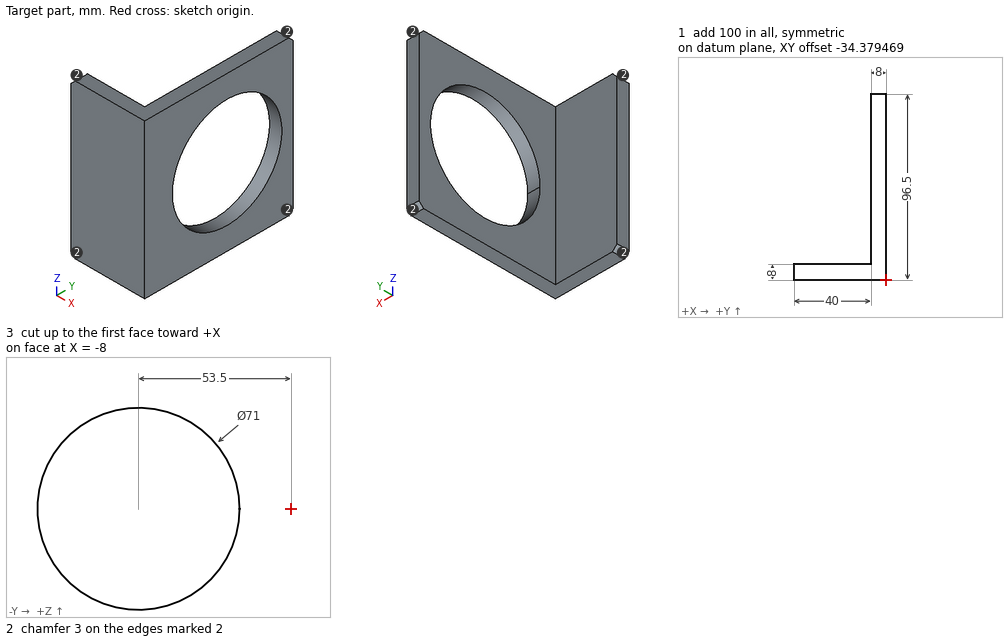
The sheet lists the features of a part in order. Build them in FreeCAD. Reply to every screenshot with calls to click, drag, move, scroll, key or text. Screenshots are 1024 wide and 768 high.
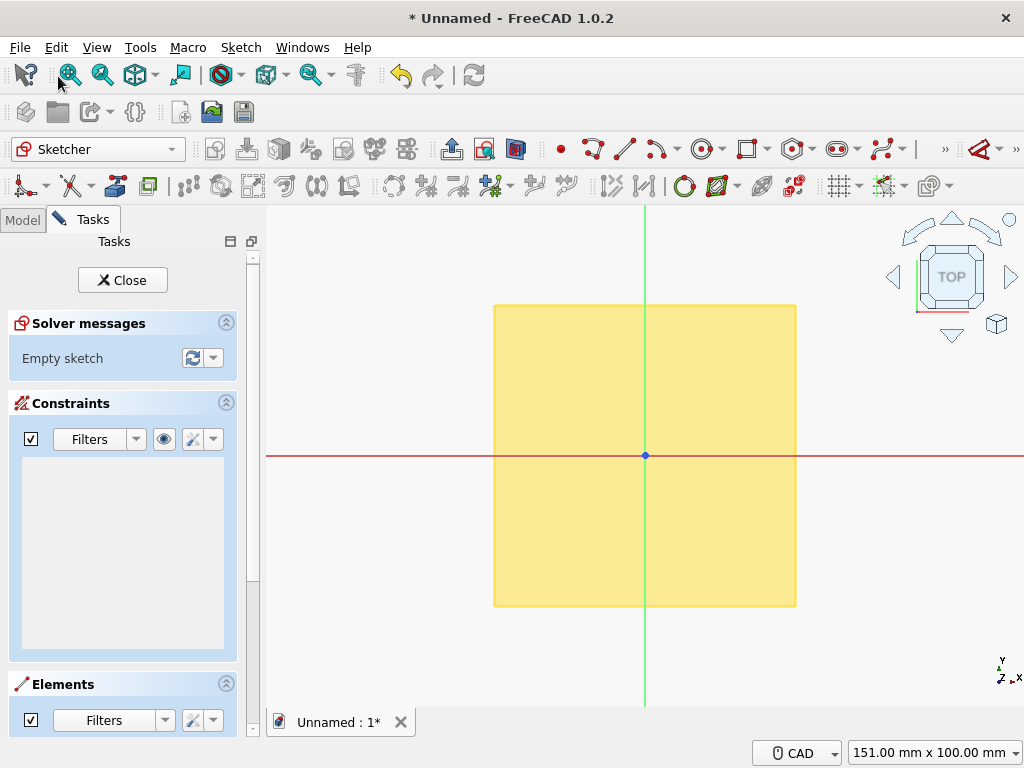
scroll(640, 679, down, 3)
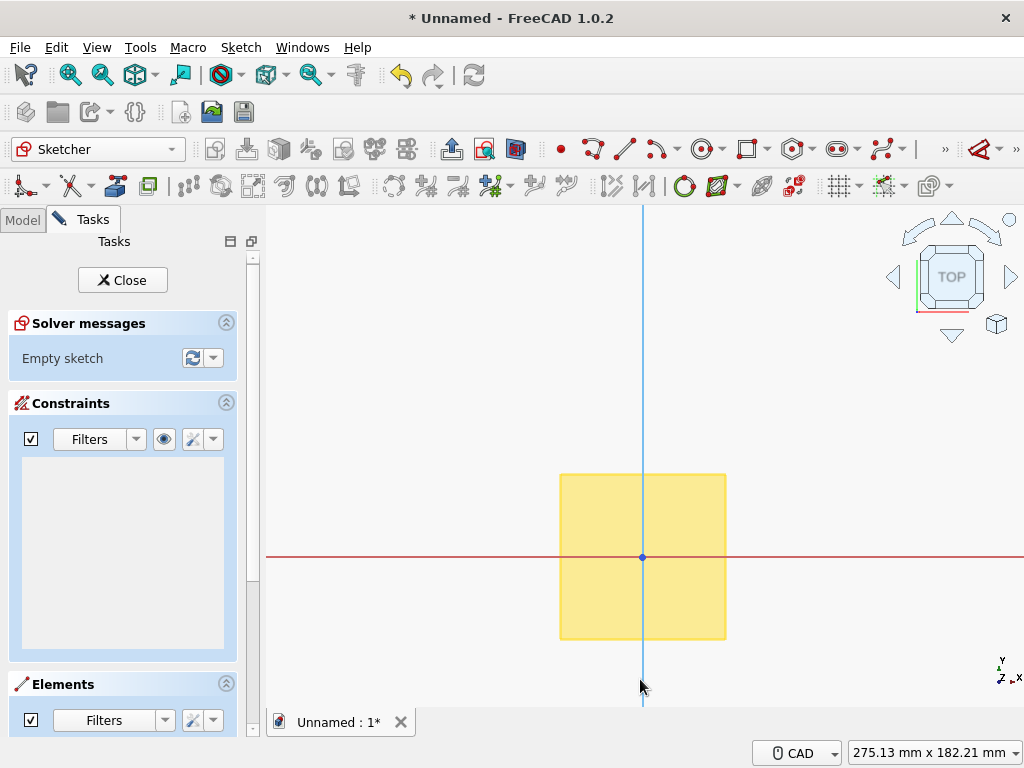
key(g)
key(m)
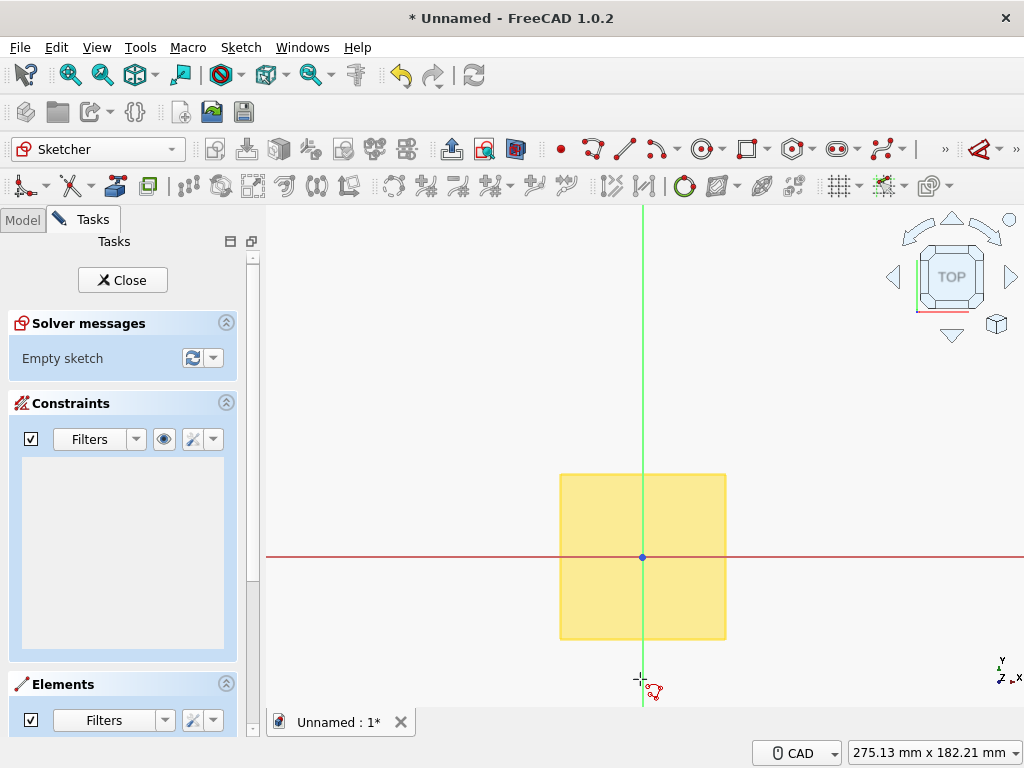
click(643, 557)
click(634, 291)
click(621, 291)
click(621, 535)
click(511, 535)
click(511, 548)
click(643, 557)
key(Escape)
key(Escape)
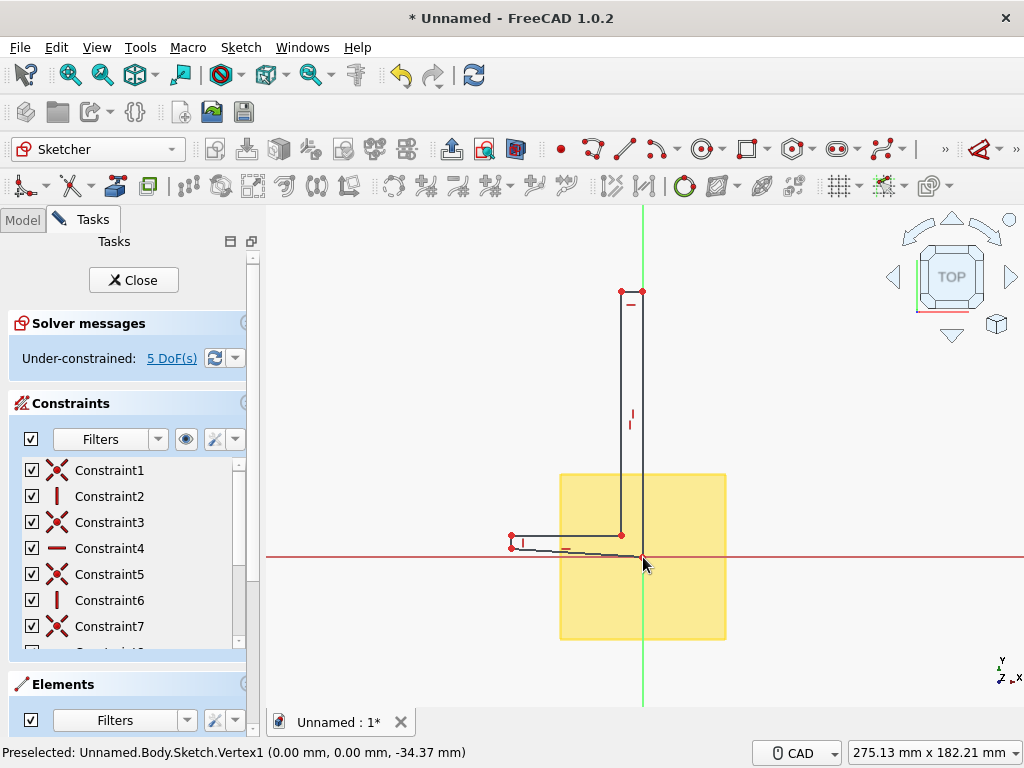
click(603, 555)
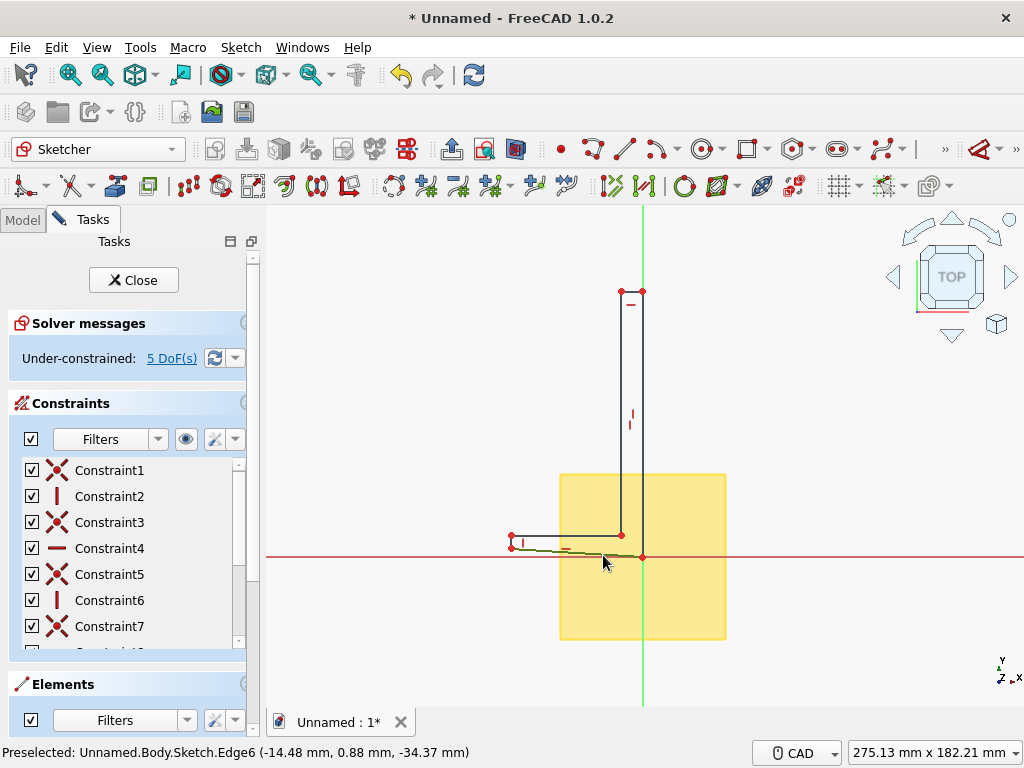
key(h)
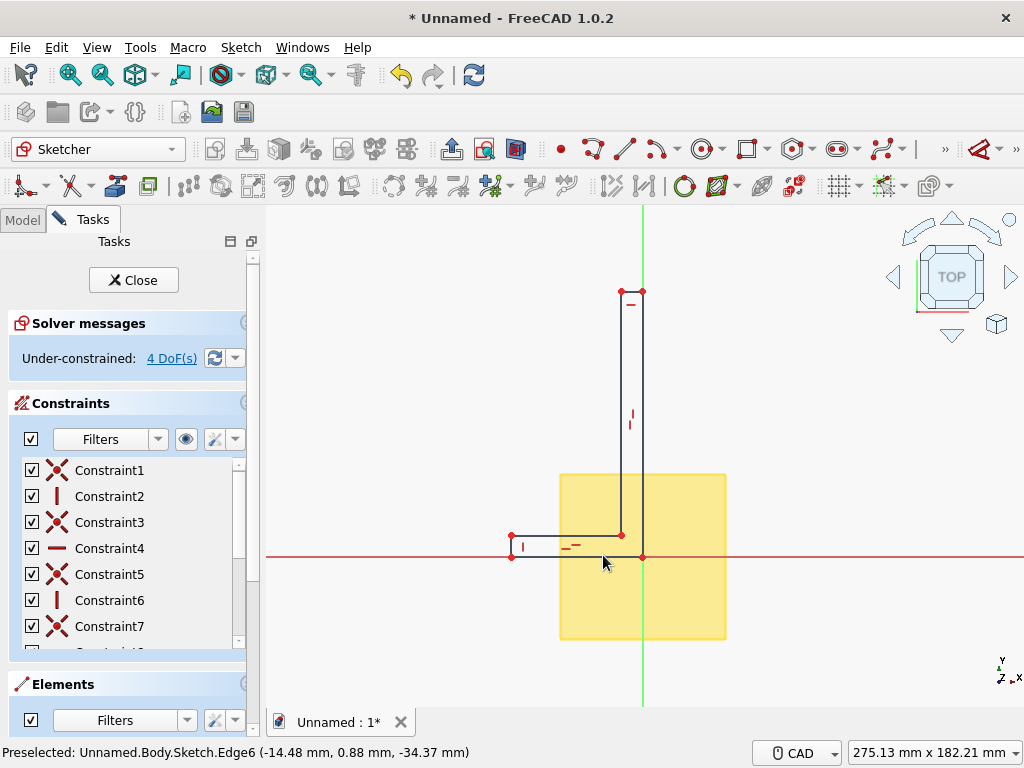
click(980, 150)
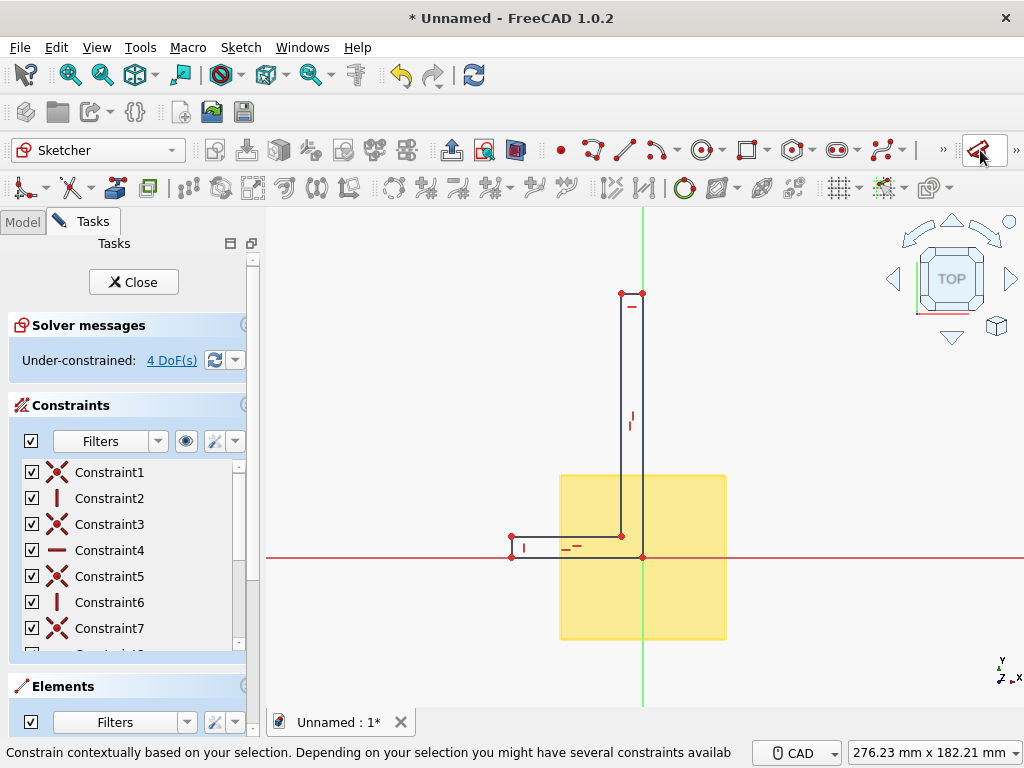
scroll(632, 294, up, 3)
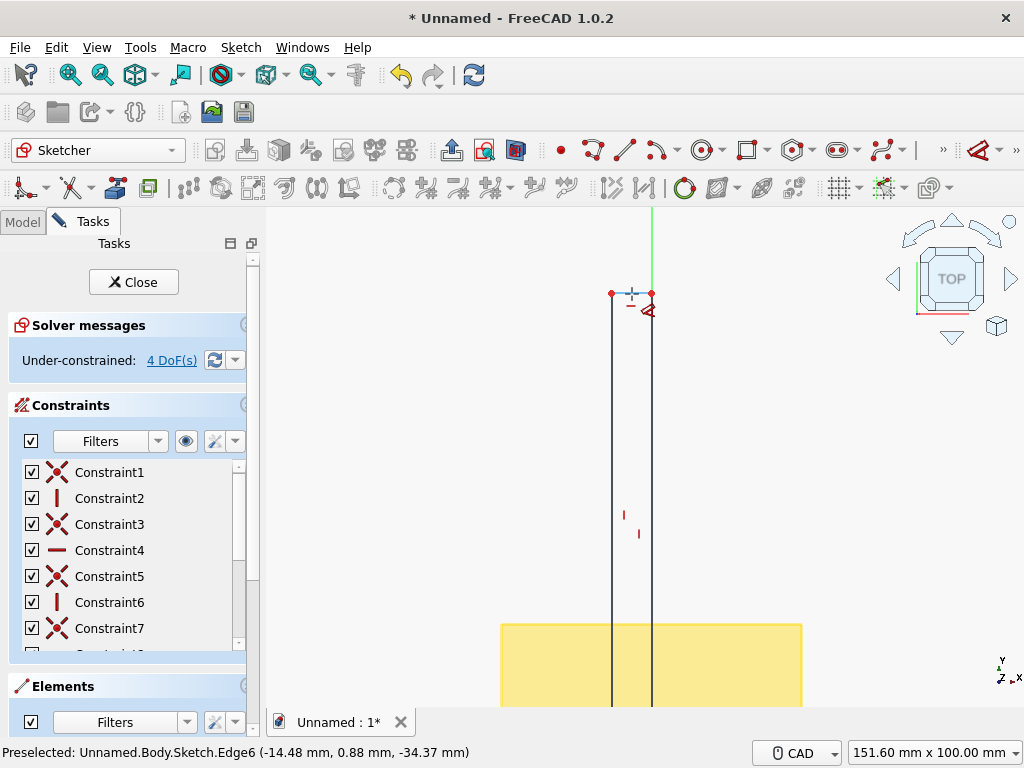
click(632, 293)
click(632, 259)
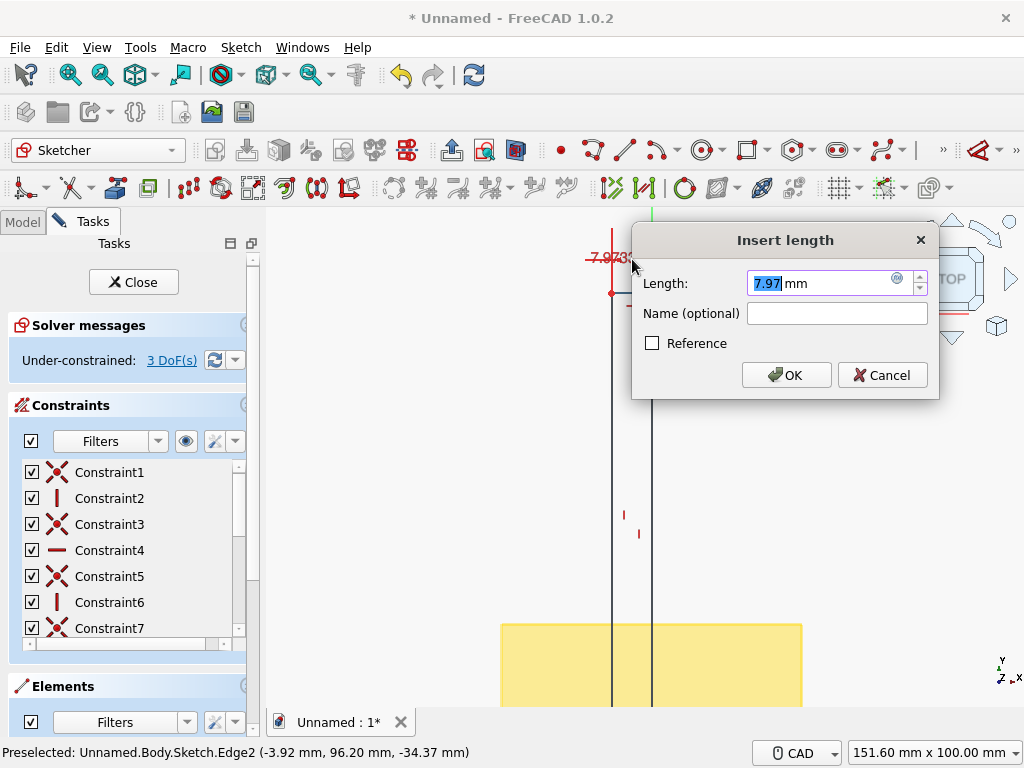
text(8)
key(Return)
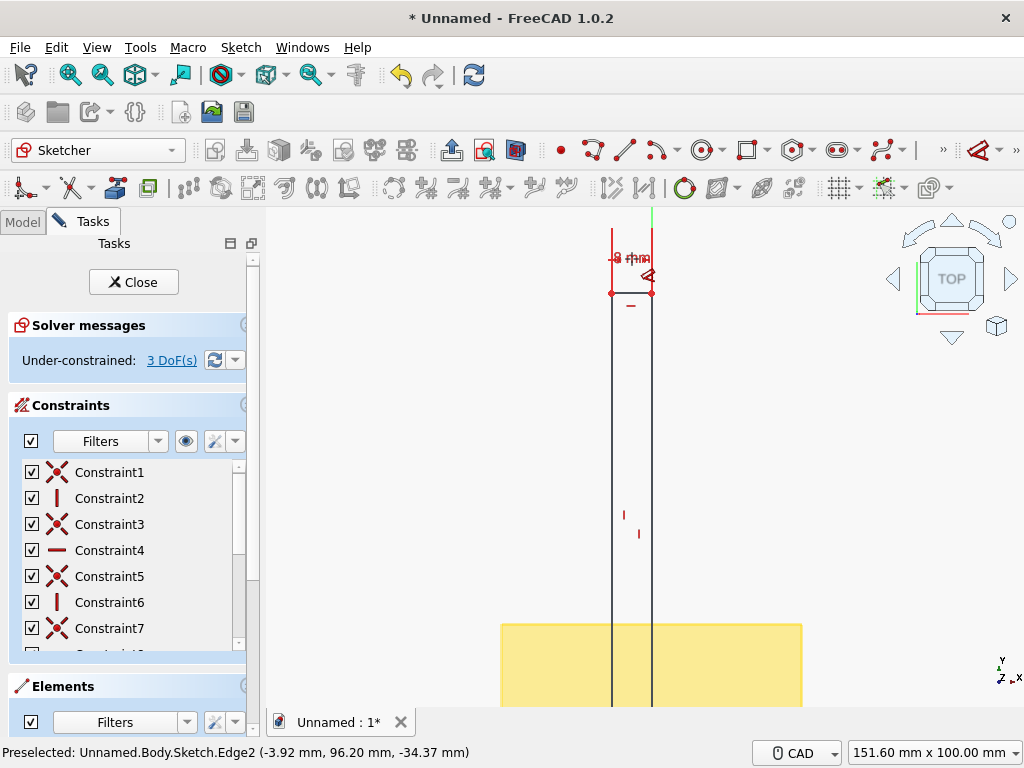
scroll(668, 302, down, 2)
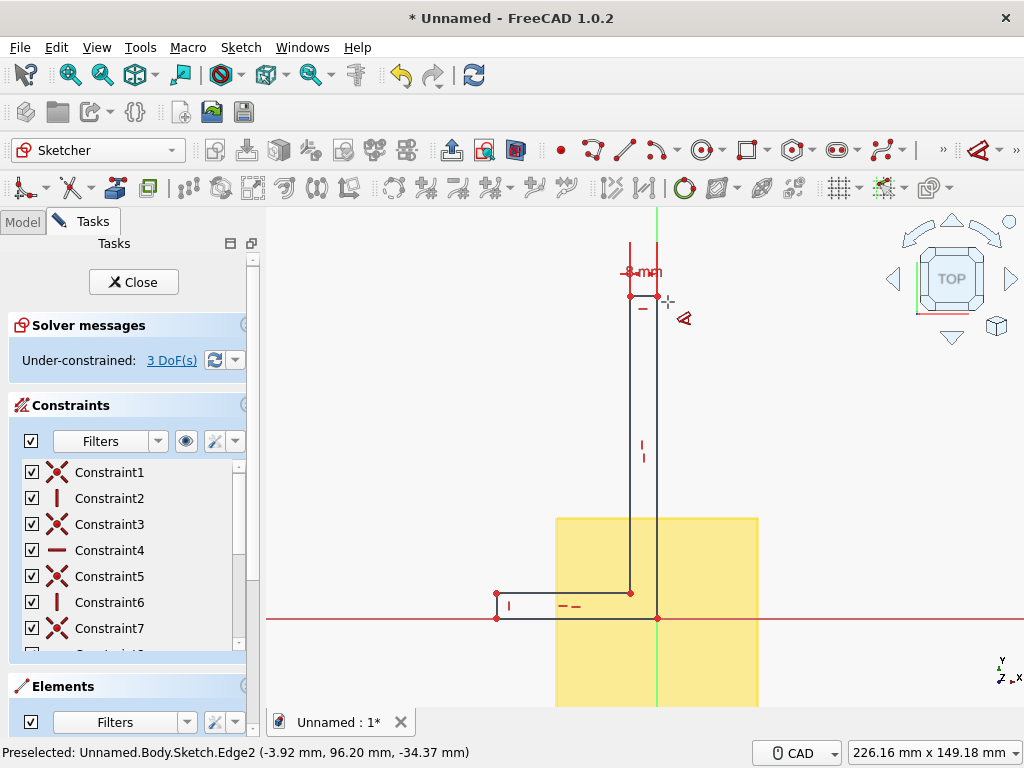
scroll(497, 601, up, 3)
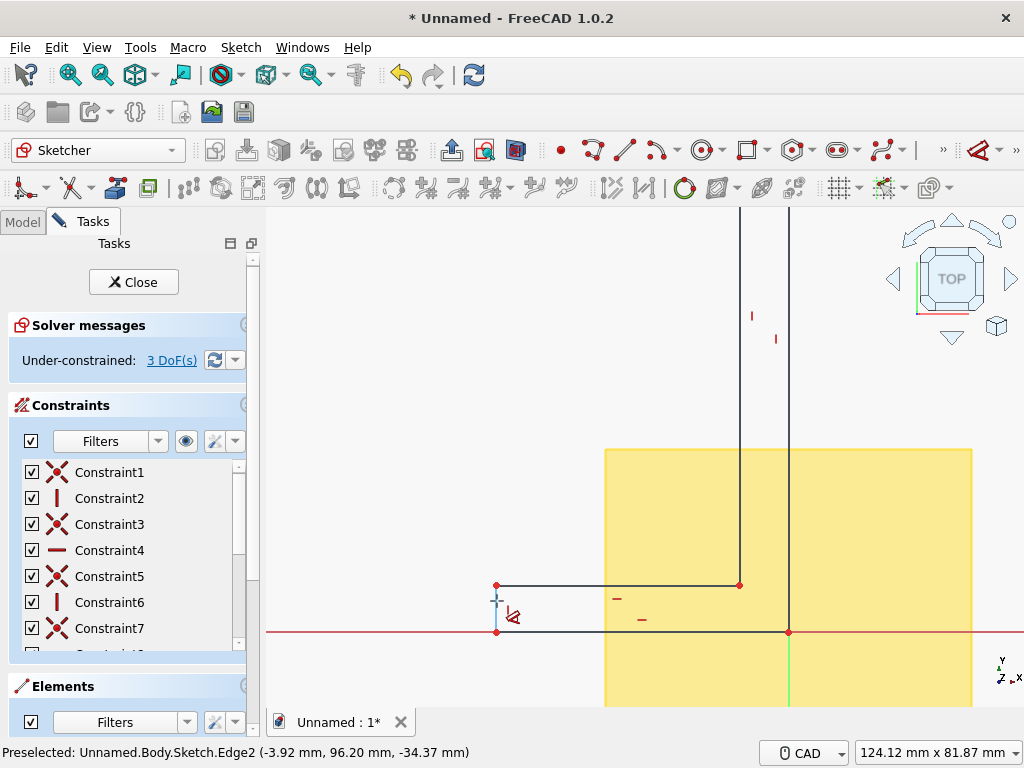
click(496, 600)
click(462, 609)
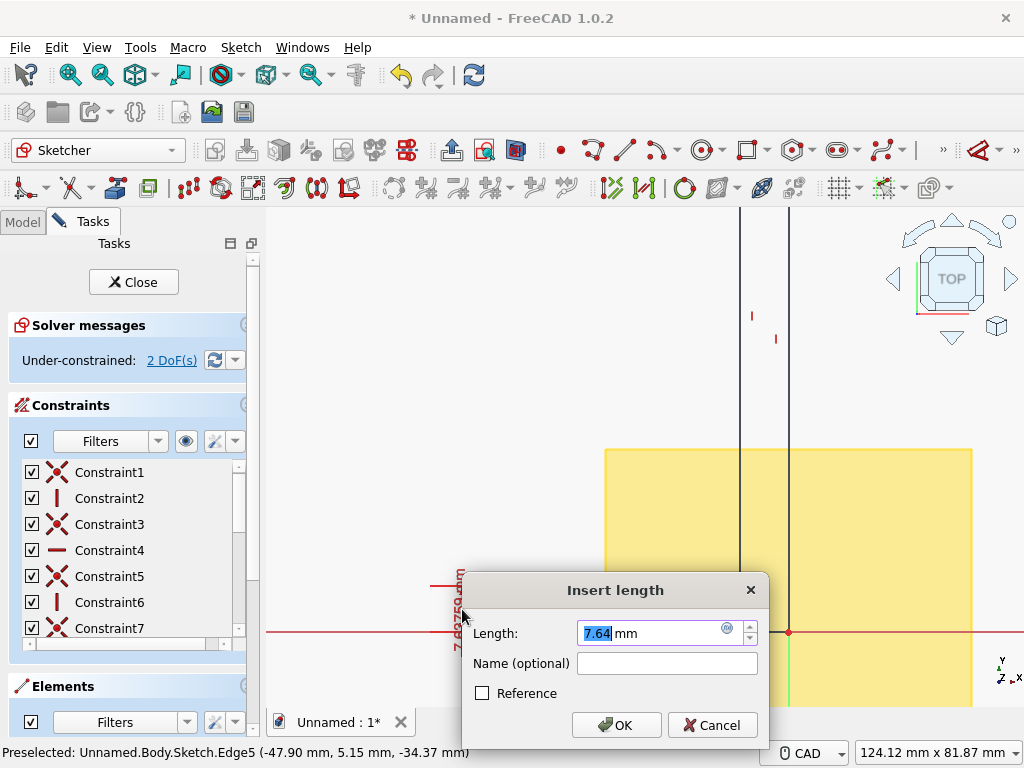
text(8)
key(Return)